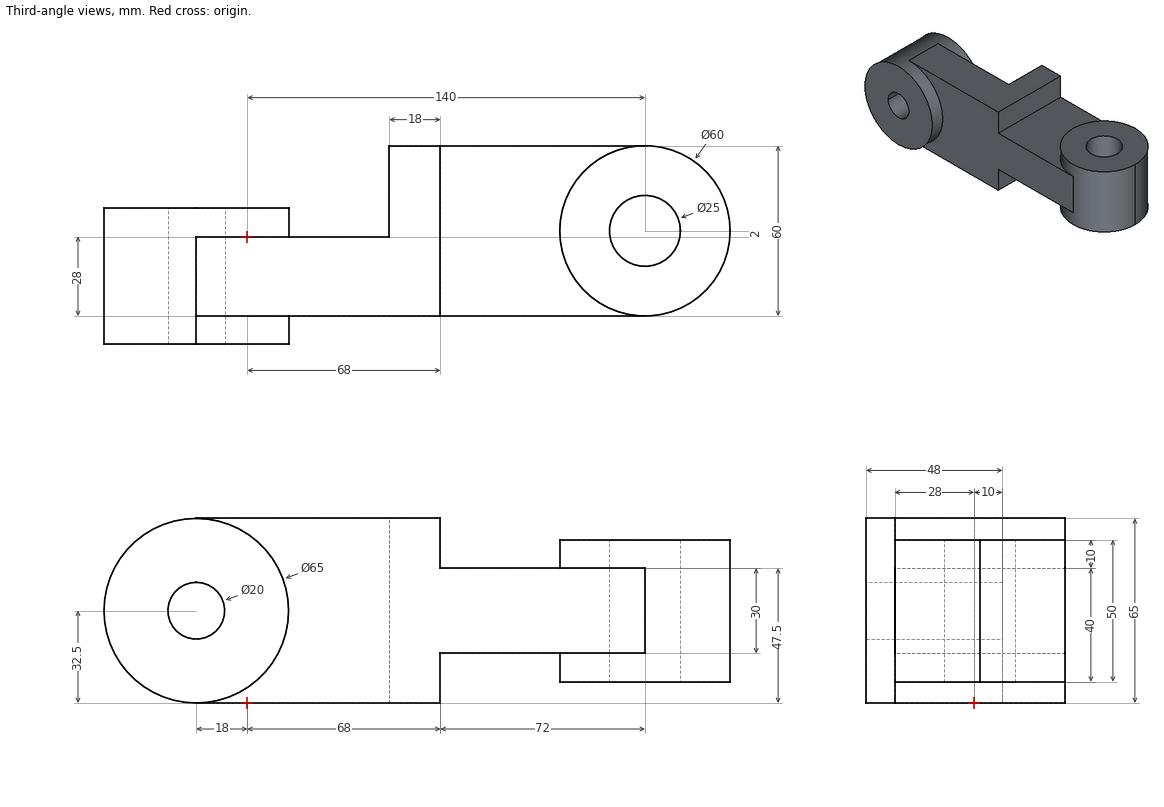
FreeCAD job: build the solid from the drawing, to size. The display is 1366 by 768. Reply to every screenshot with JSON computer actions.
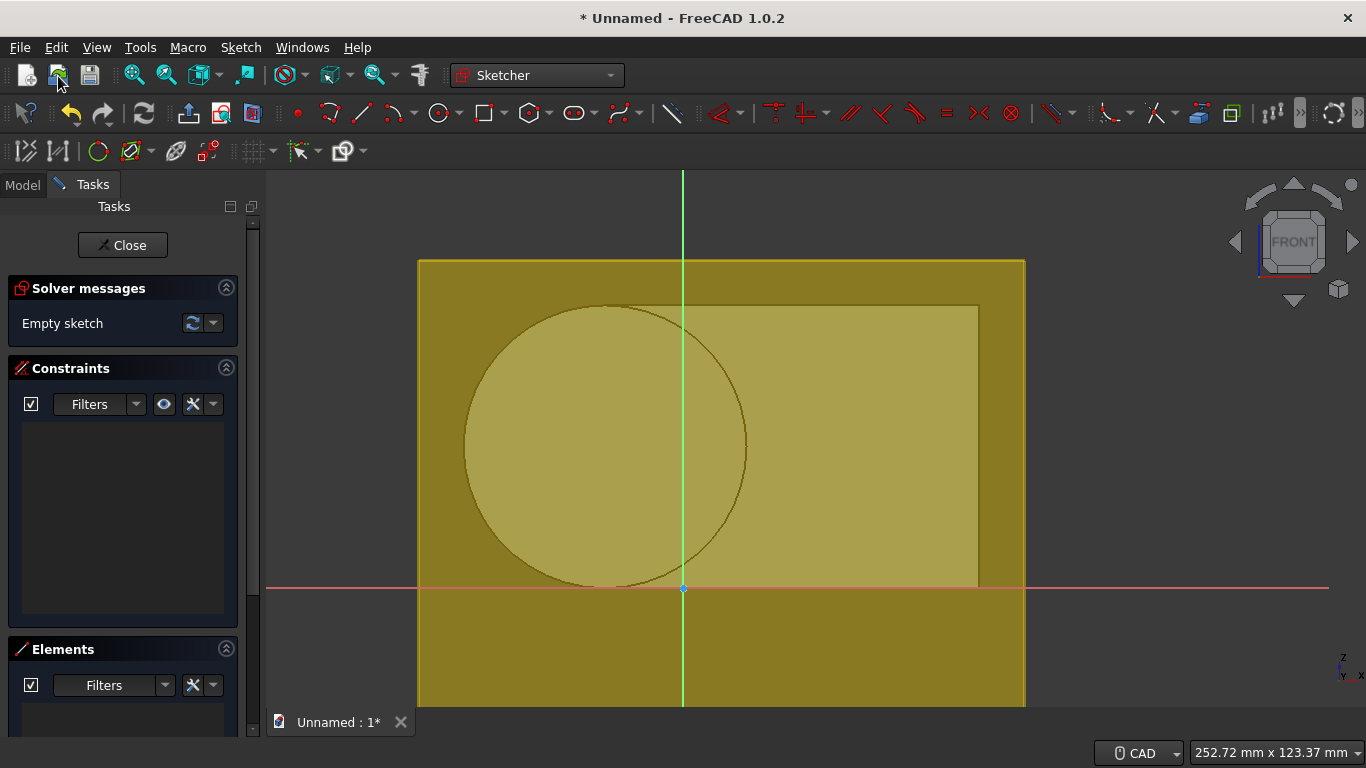
{"action": "left_click", "coordinate": [440, 114]}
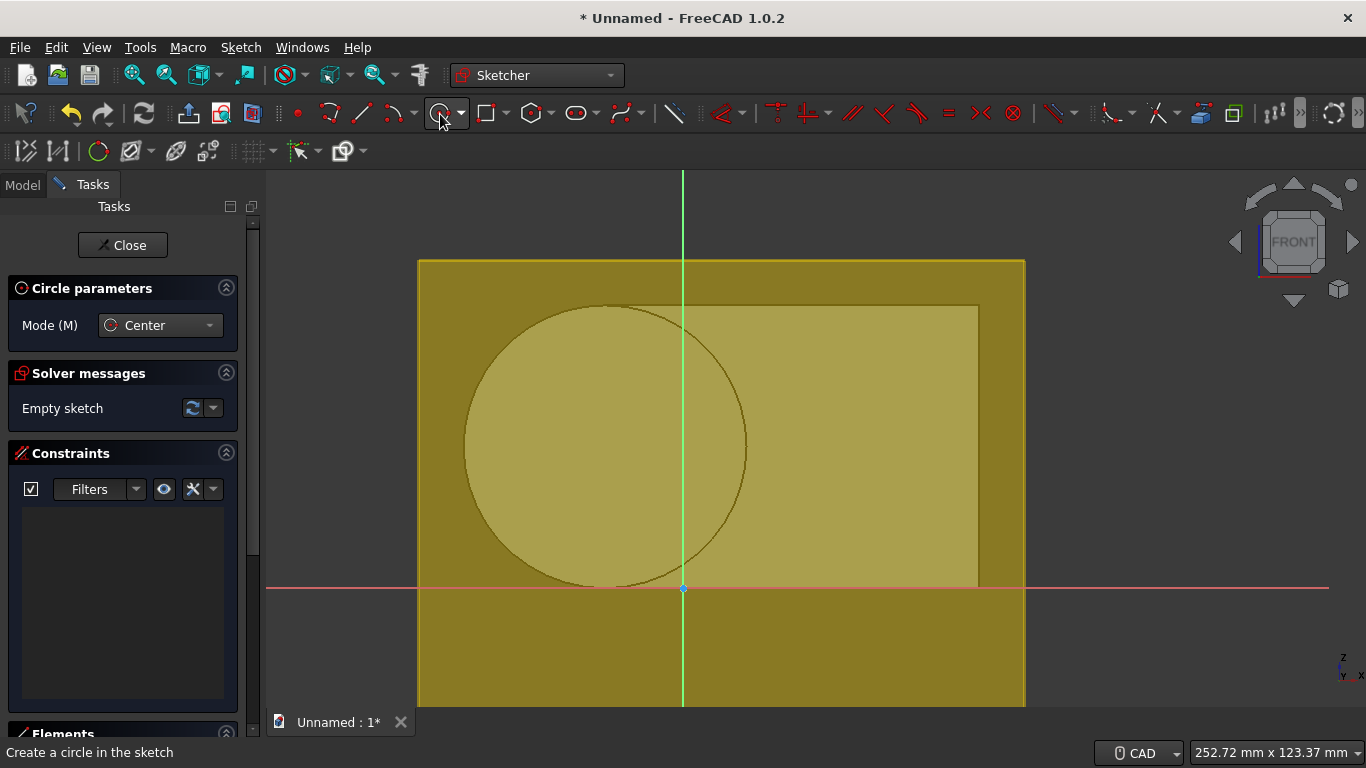
{"action": "left_click", "coordinate": [605, 447]}
{"action": "left_click", "coordinate": [705, 347]}
{"action": "key", "text": "Escape"}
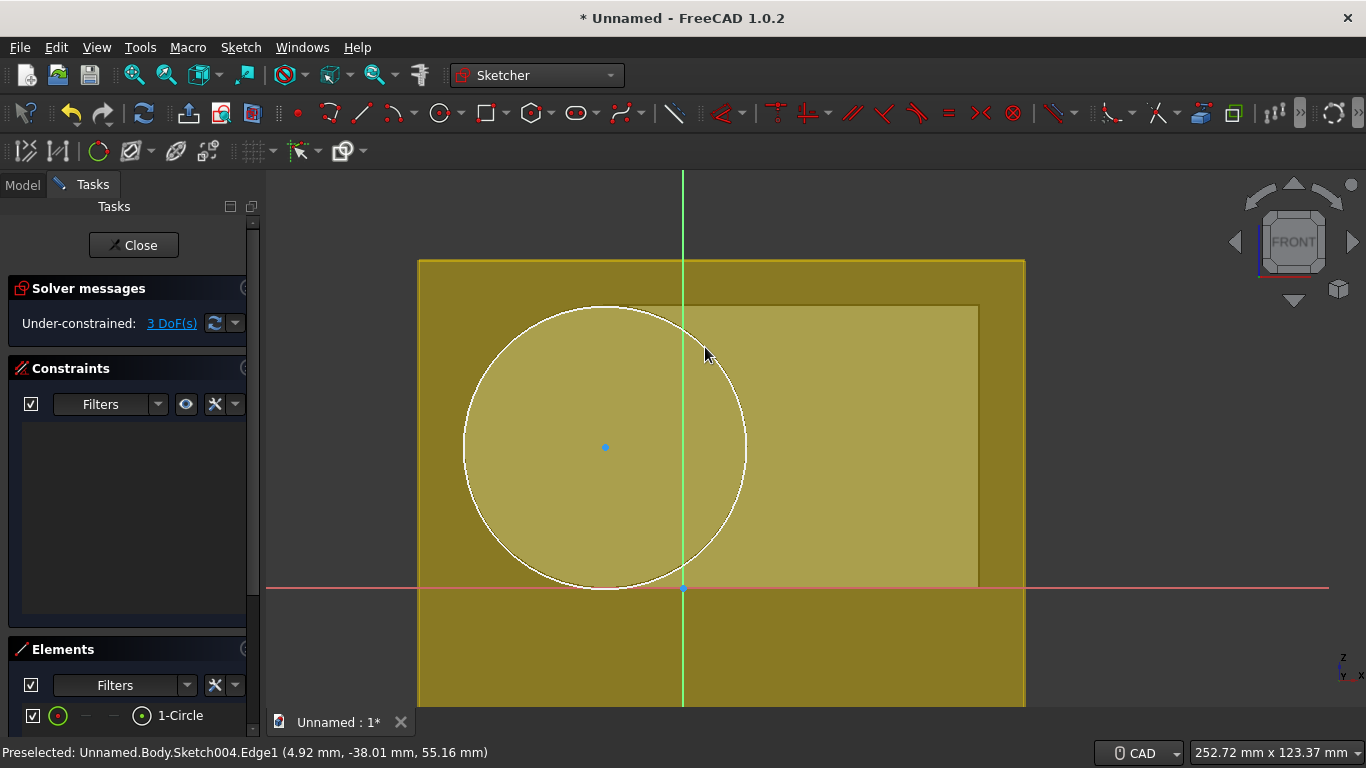
{"action": "left_click", "coordinate": [722, 114]}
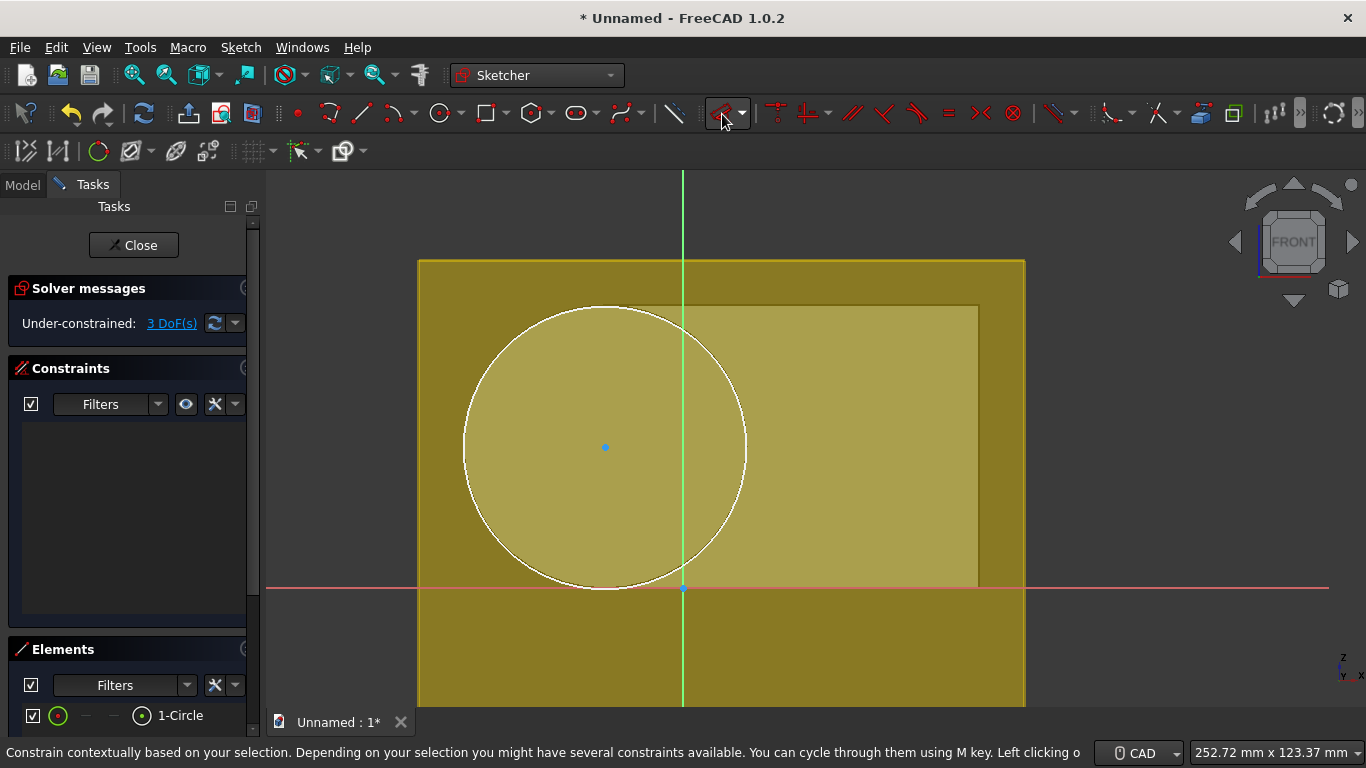
{"action": "left_click", "coordinate": [705, 348]}
{"action": "left_click", "coordinate": [728, 325]}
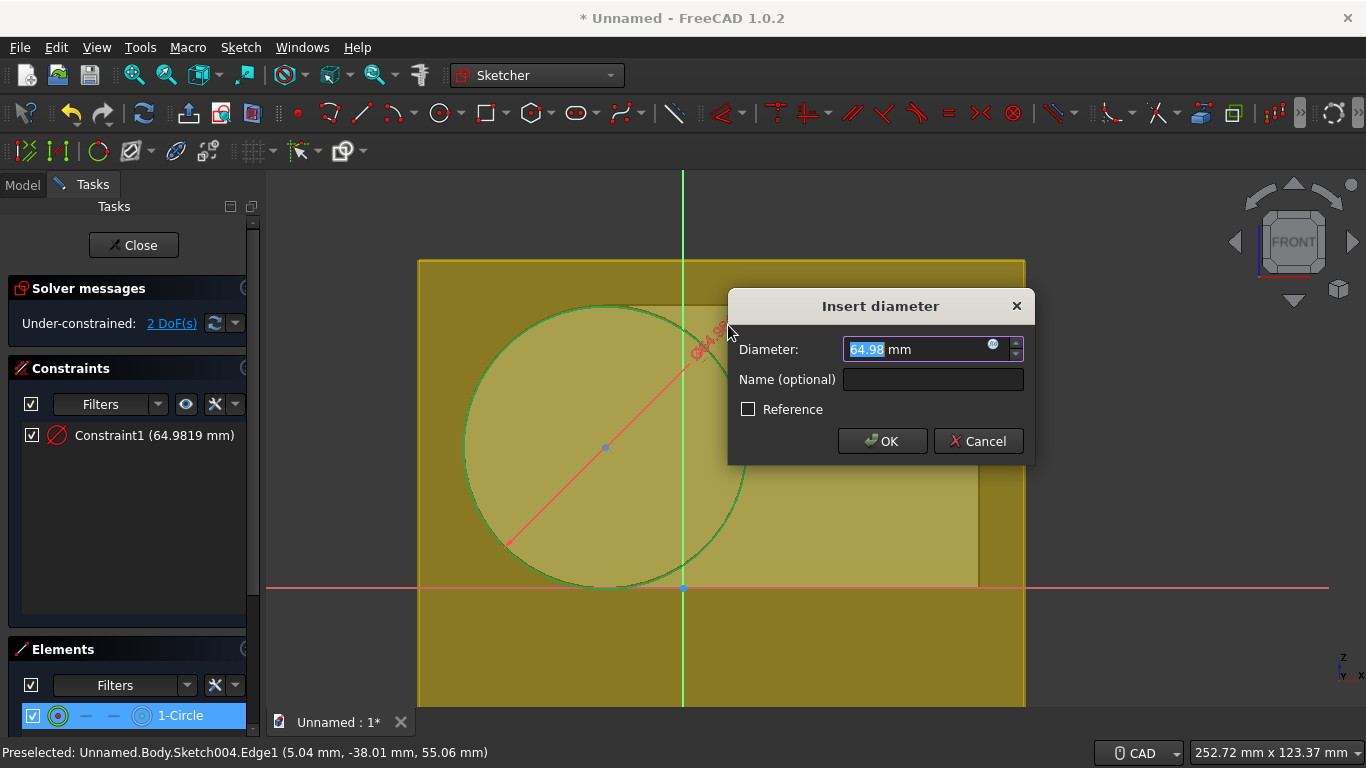
{"action": "type", "text": "65"}
{"action": "key", "text": "Return"}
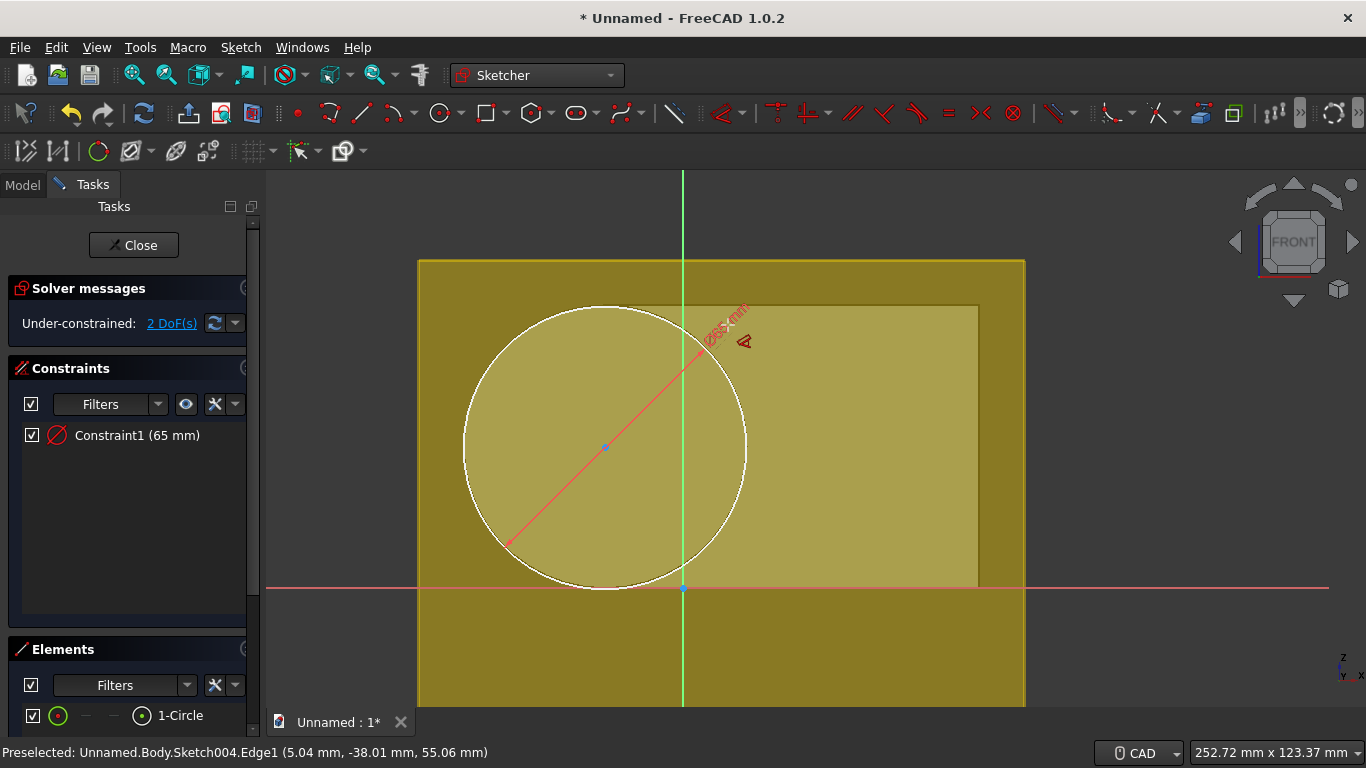
{"action": "left_click", "coordinate": [605, 448]}
{"action": "left_click", "coordinate": [644, 622]}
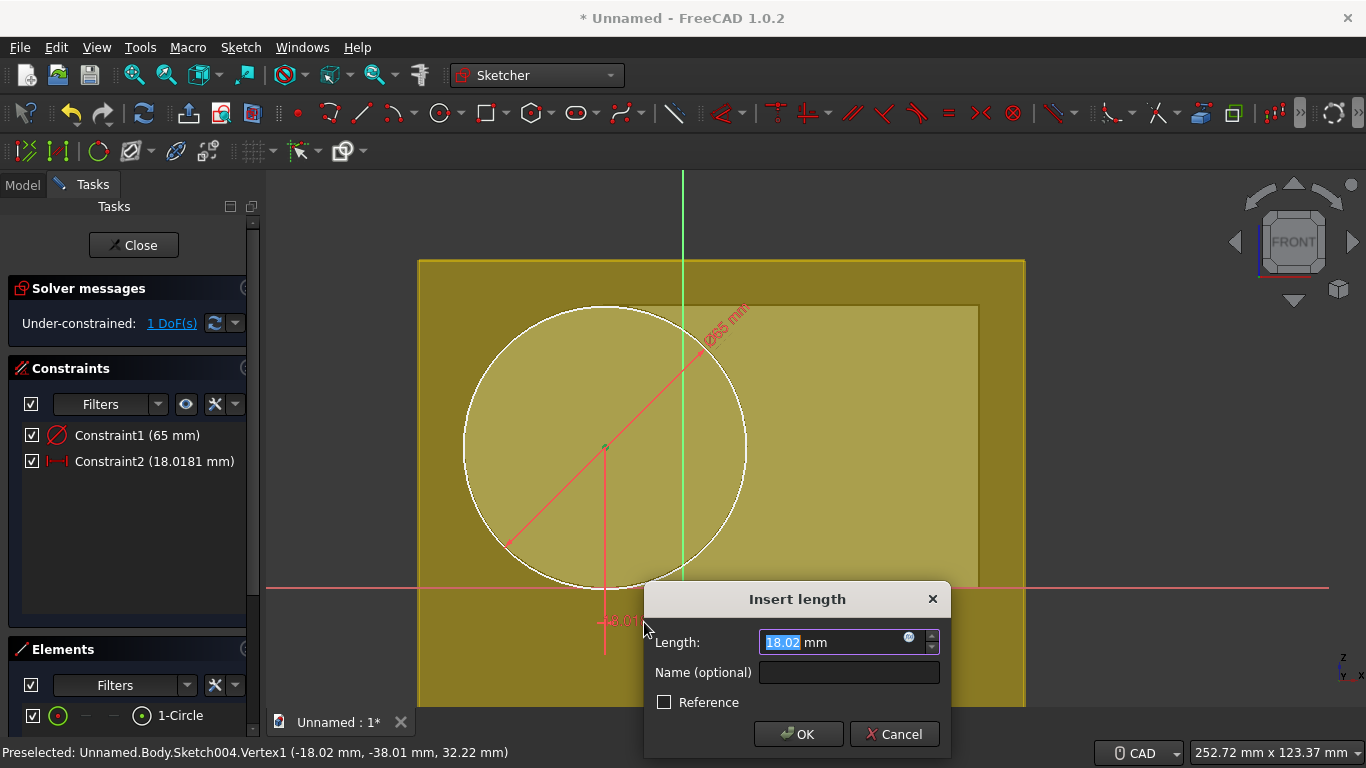
{"action": "type", "text": "18"}
{"action": "key", "text": "Return"}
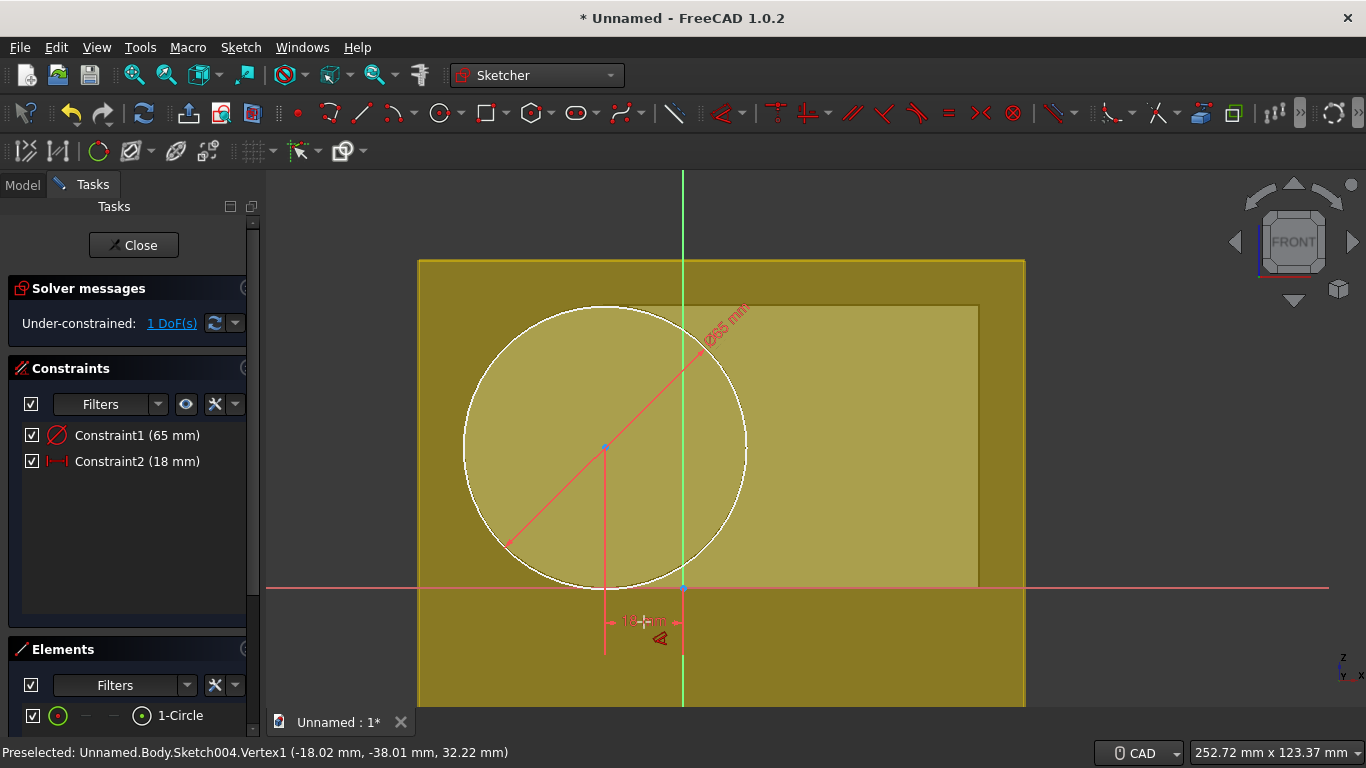
{"action": "left_click", "coordinate": [605, 448]}
{"action": "left_click", "coordinate": [717, 486]}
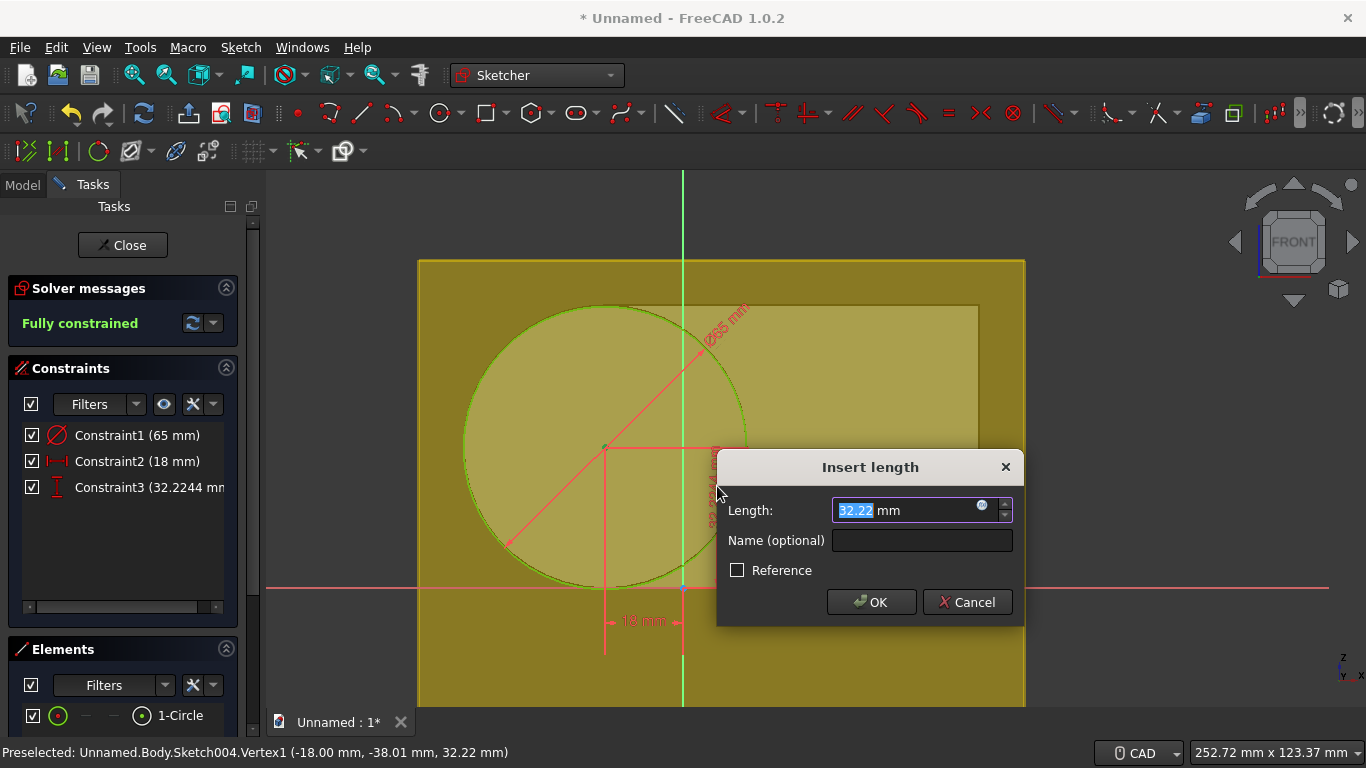
{"action": "type", "text": "32.5"}
{"action": "key", "text": "Return"}
{"action": "key", "text": "Escape"}